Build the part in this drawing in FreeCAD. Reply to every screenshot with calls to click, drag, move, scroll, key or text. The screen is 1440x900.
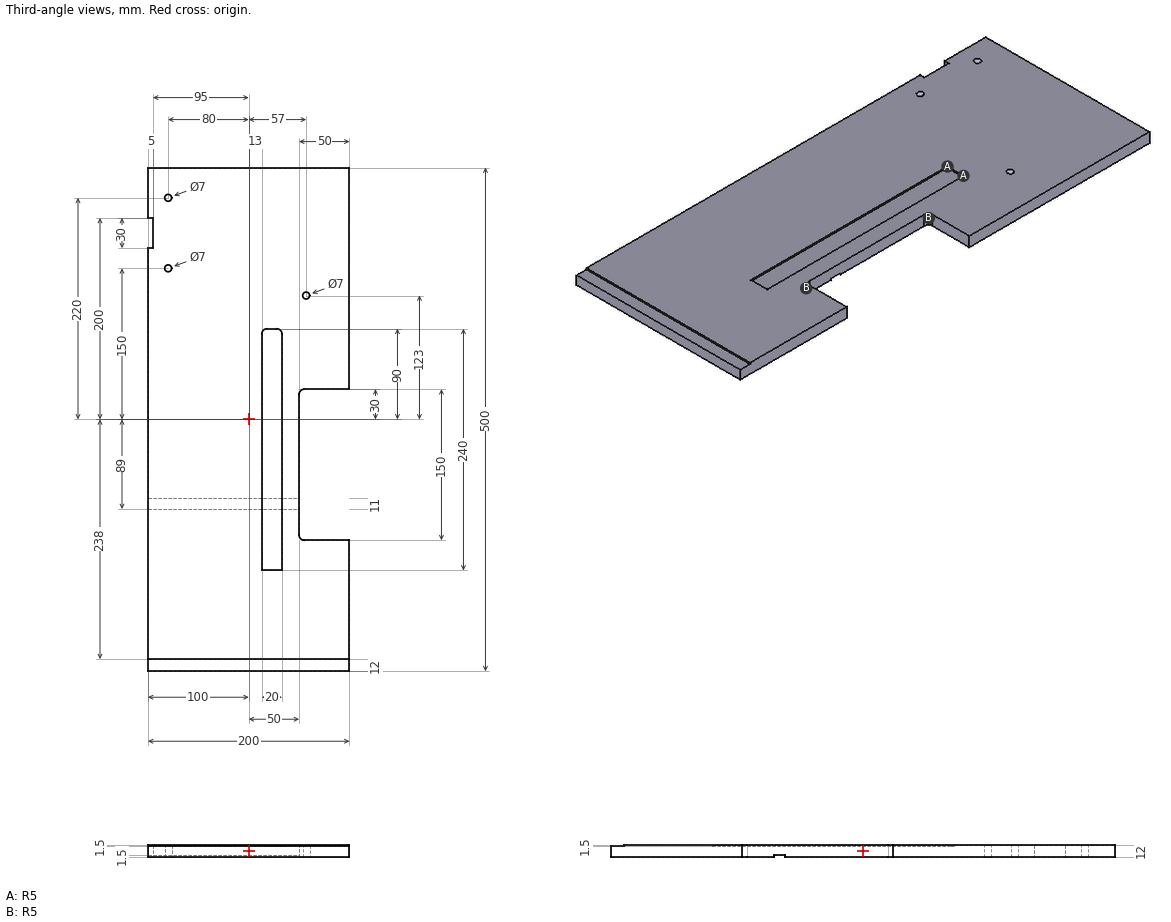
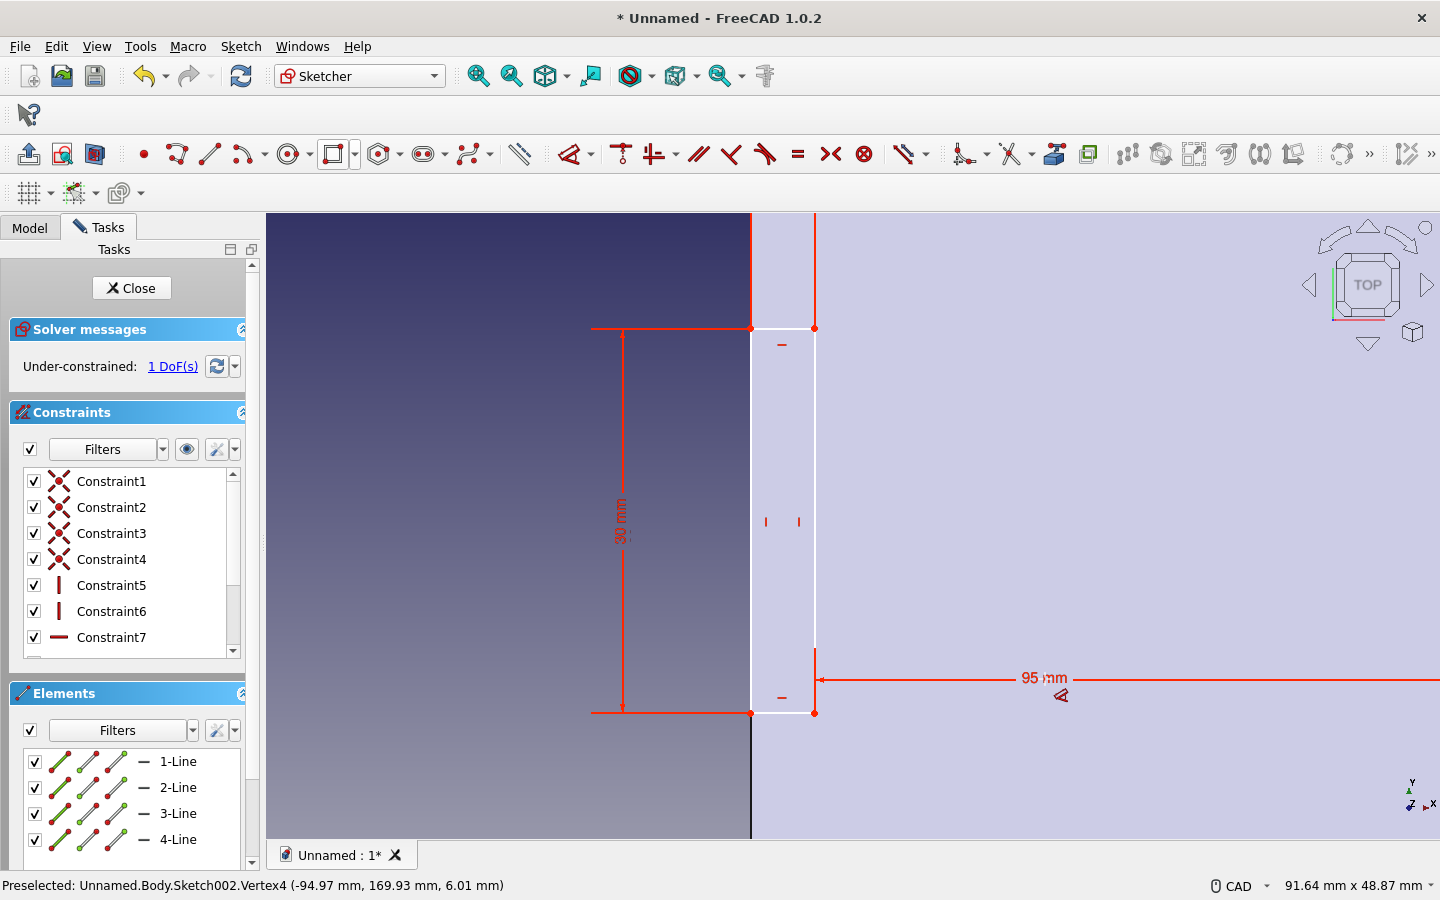
click(751, 329)
click(717, 570)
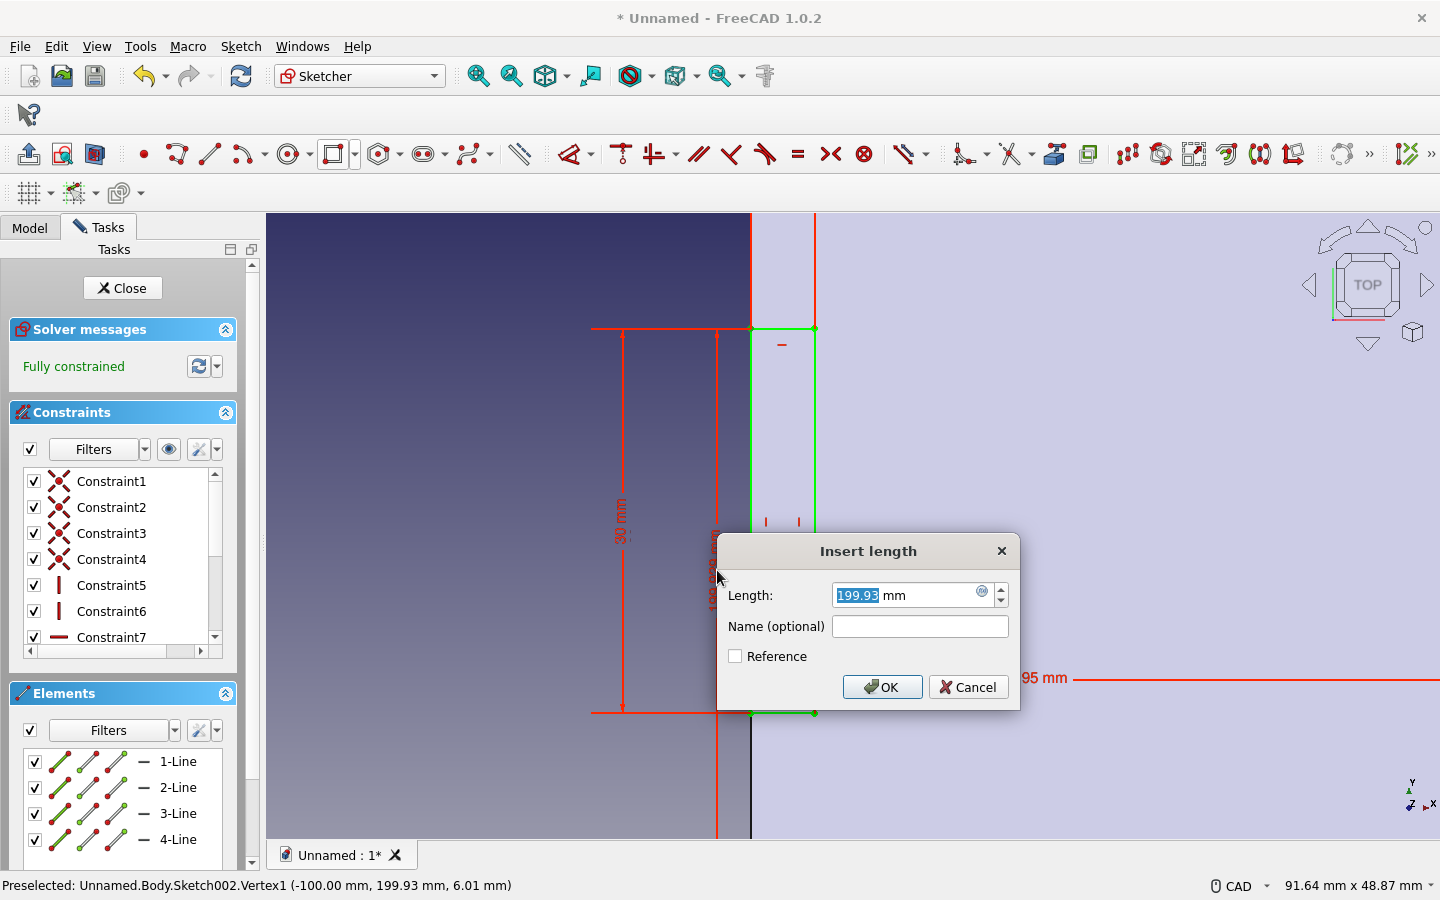
text(200)
key(Return)
key(Escape)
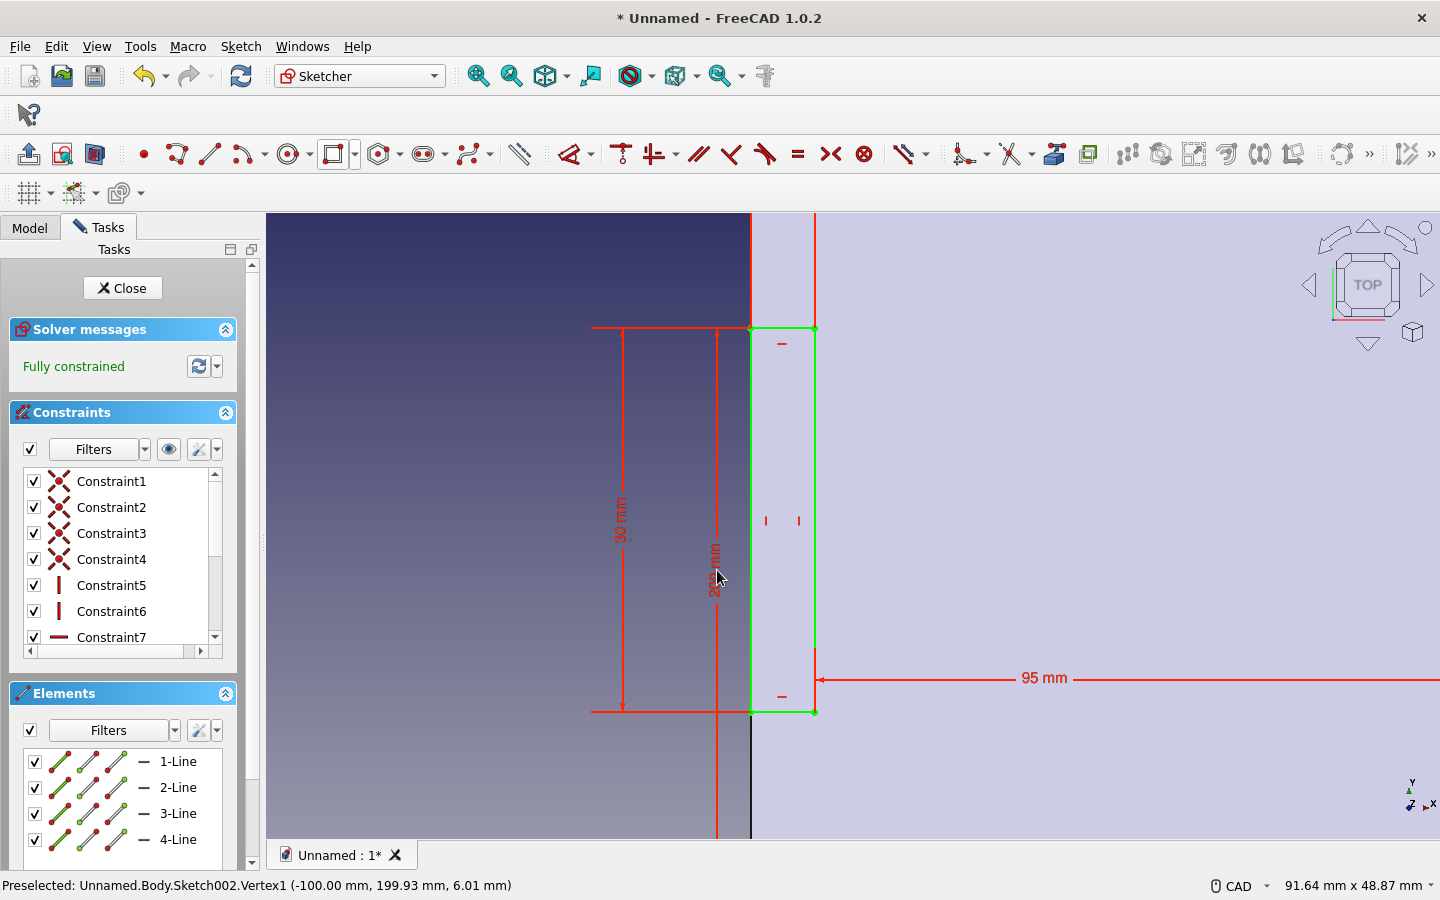
click(123, 288)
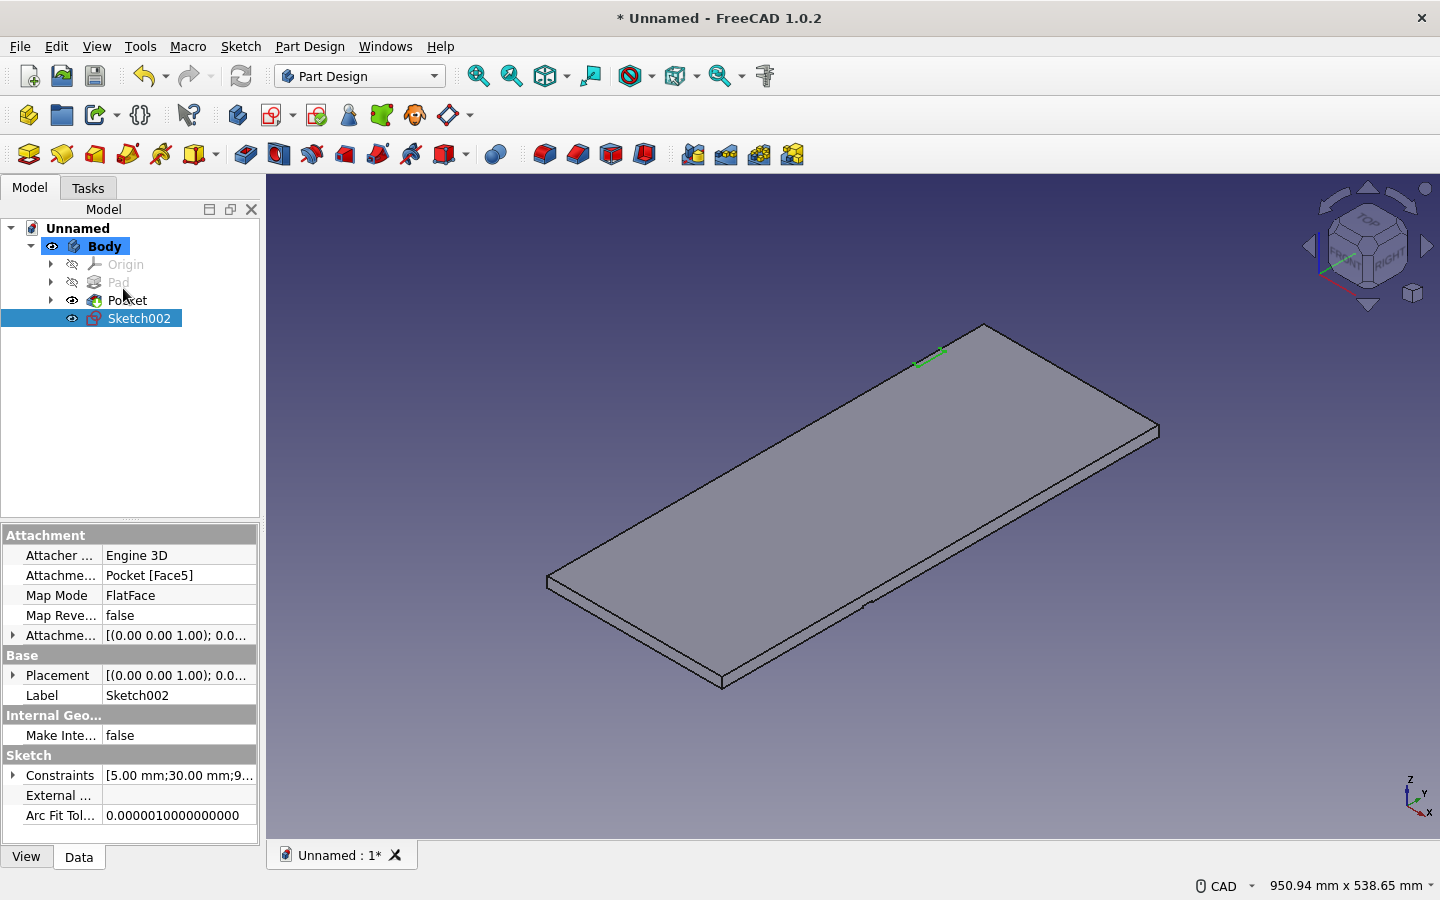
click(246, 154)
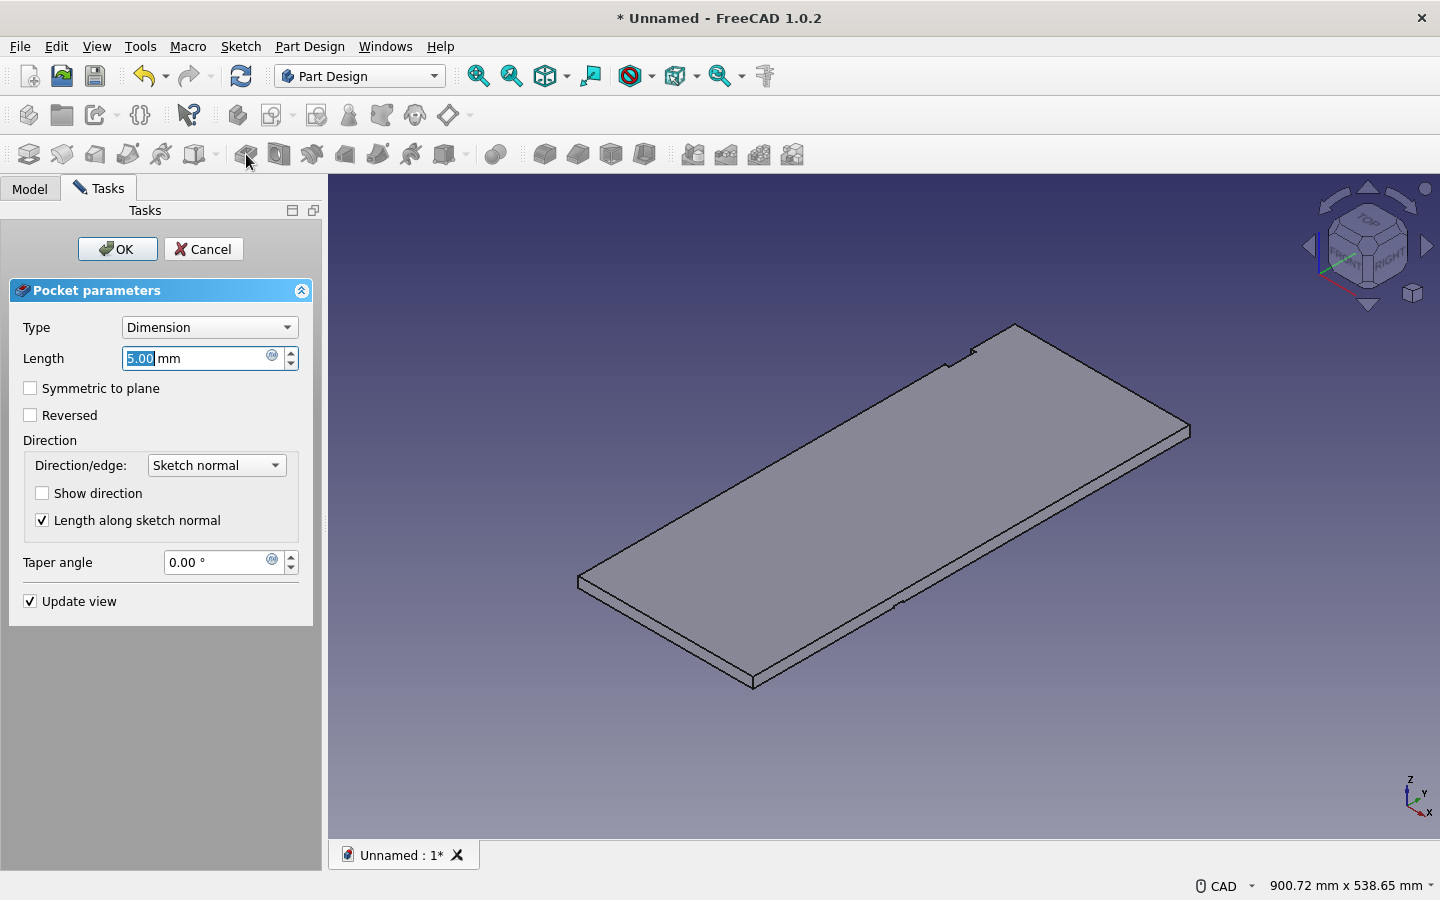
click(210, 328)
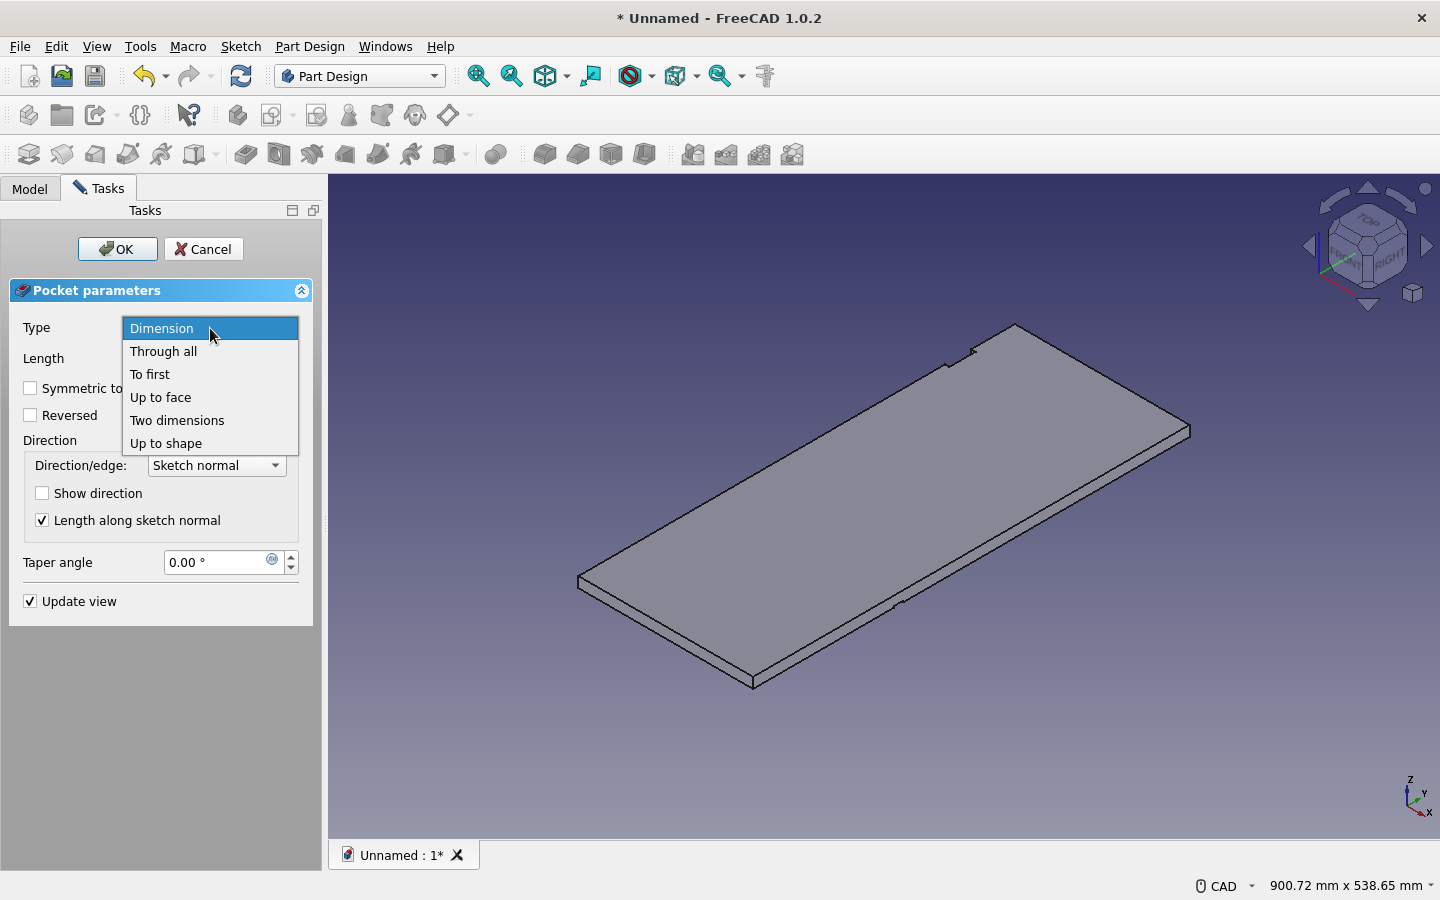
click(208, 374)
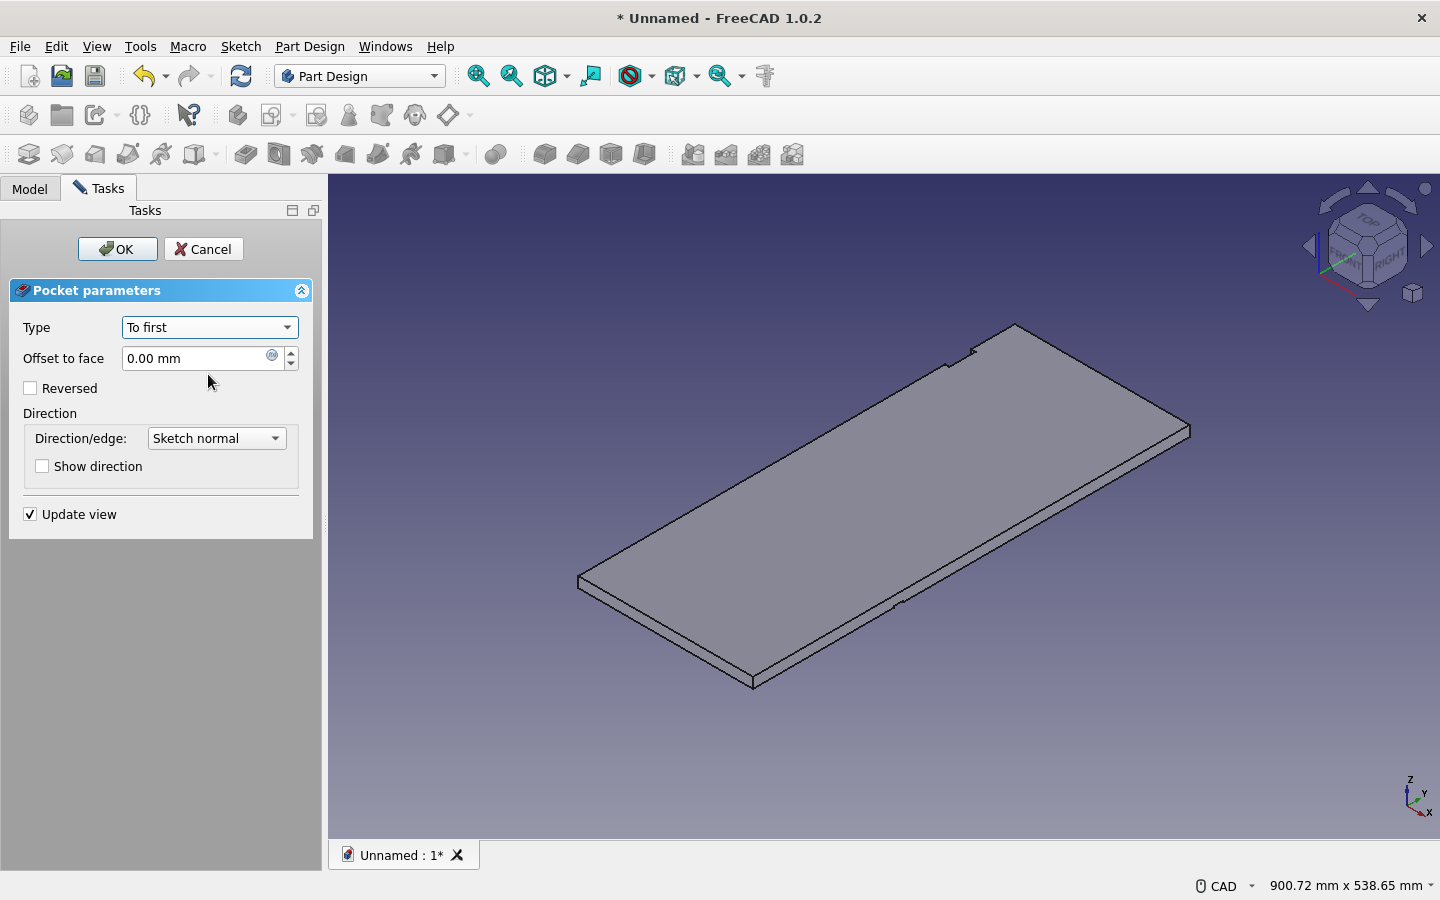
click(118, 249)